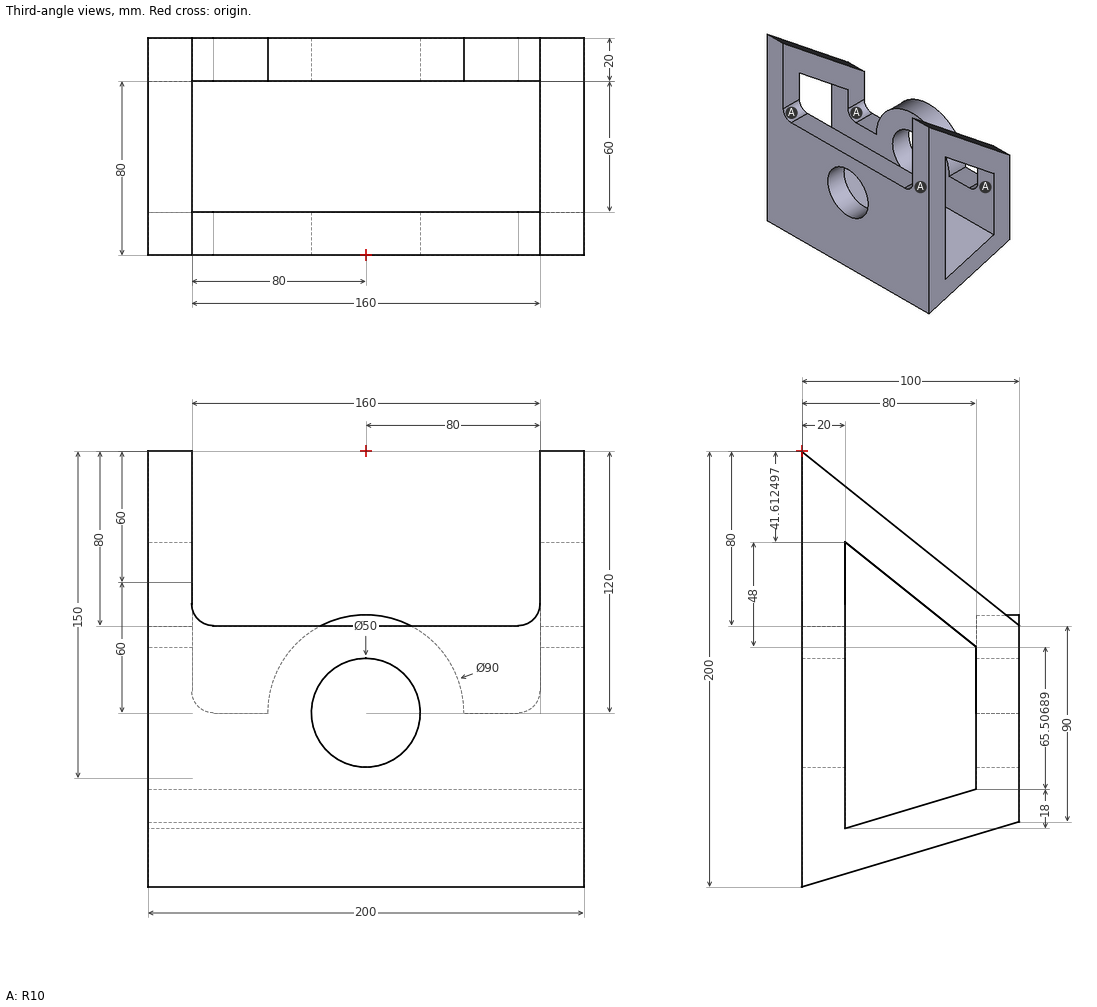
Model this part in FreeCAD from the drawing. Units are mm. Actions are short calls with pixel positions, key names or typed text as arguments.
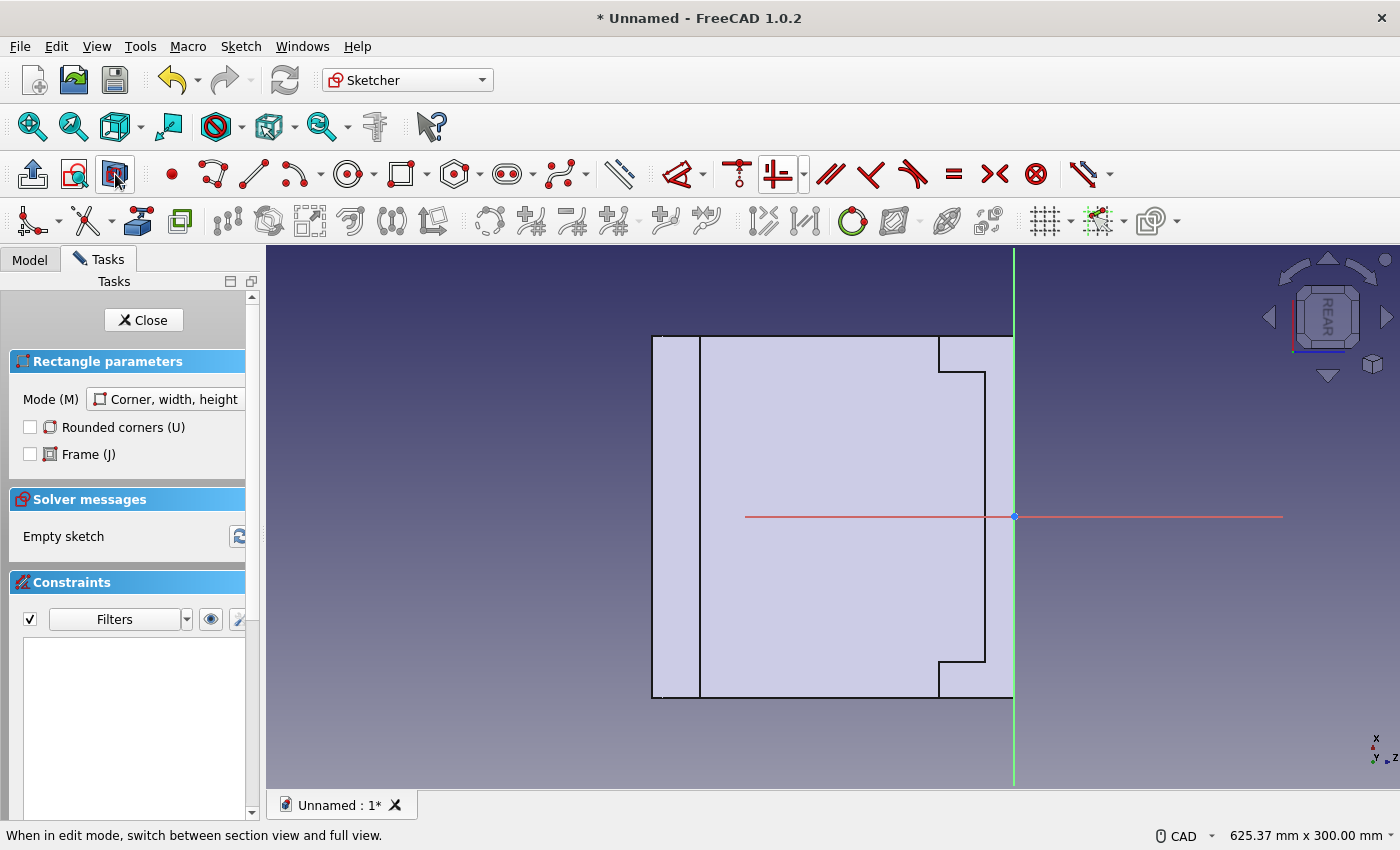
click(869, 372)
click(1014, 662)
key(Escape)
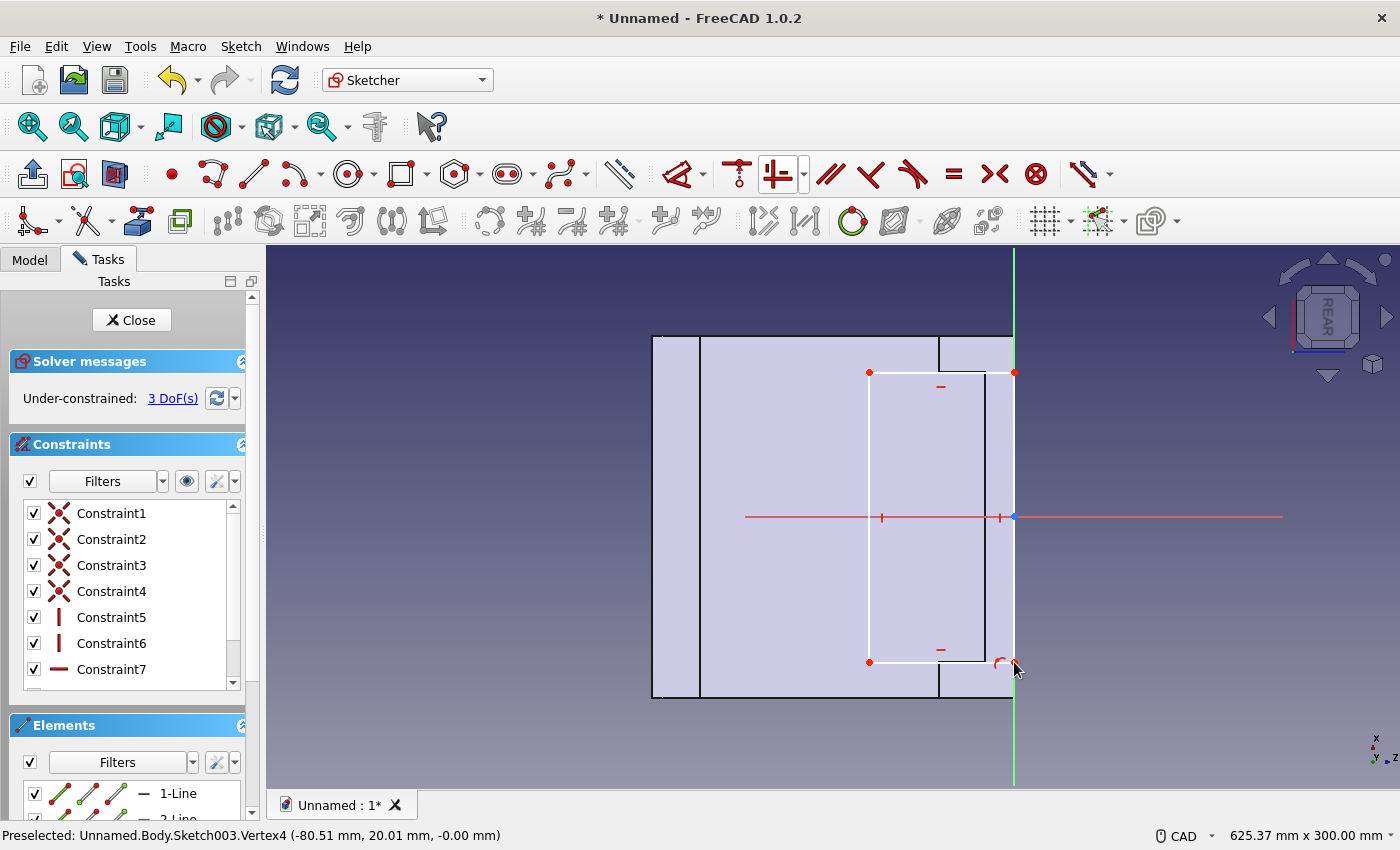
click(676, 174)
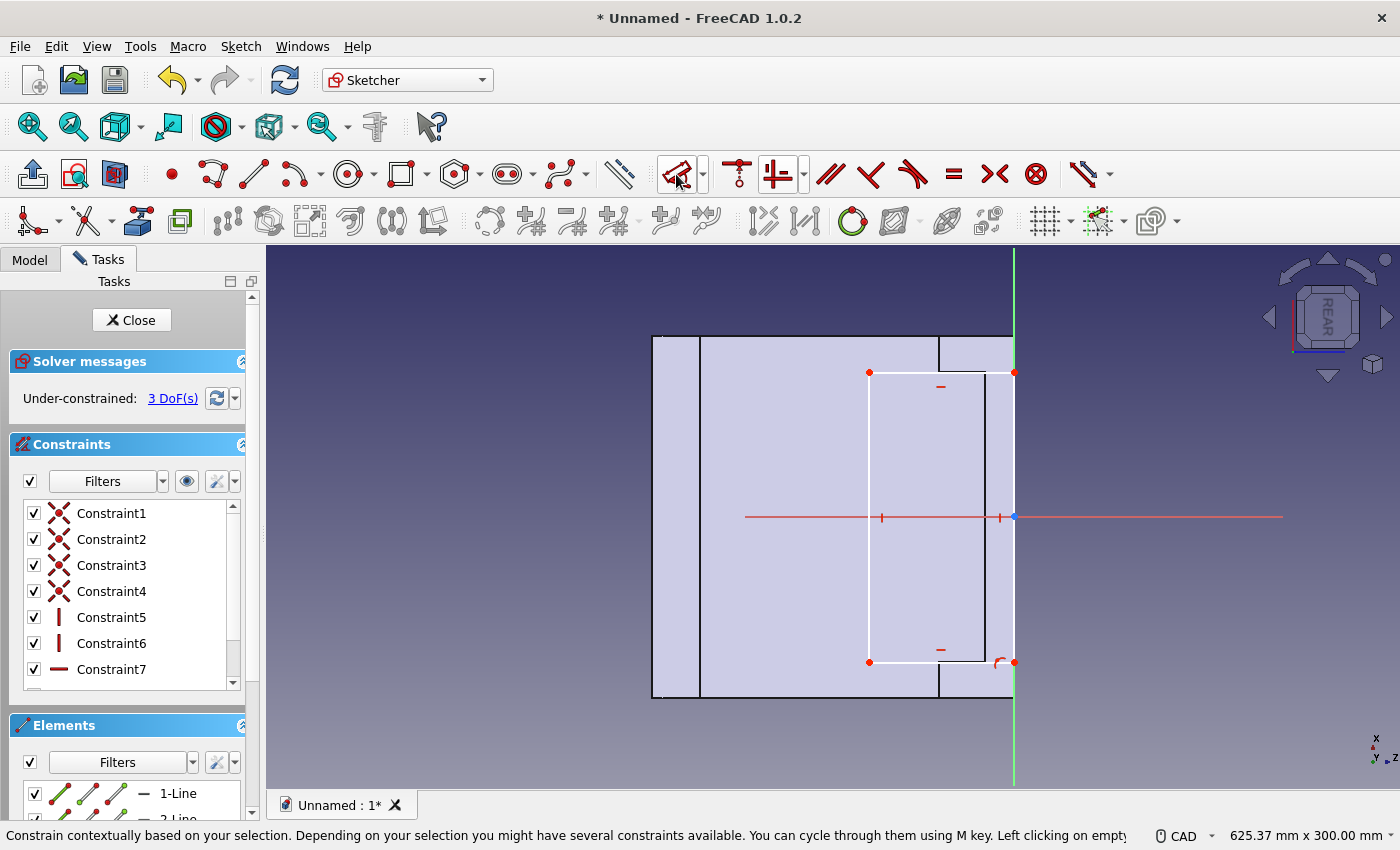
click(913, 663)
click(942, 697)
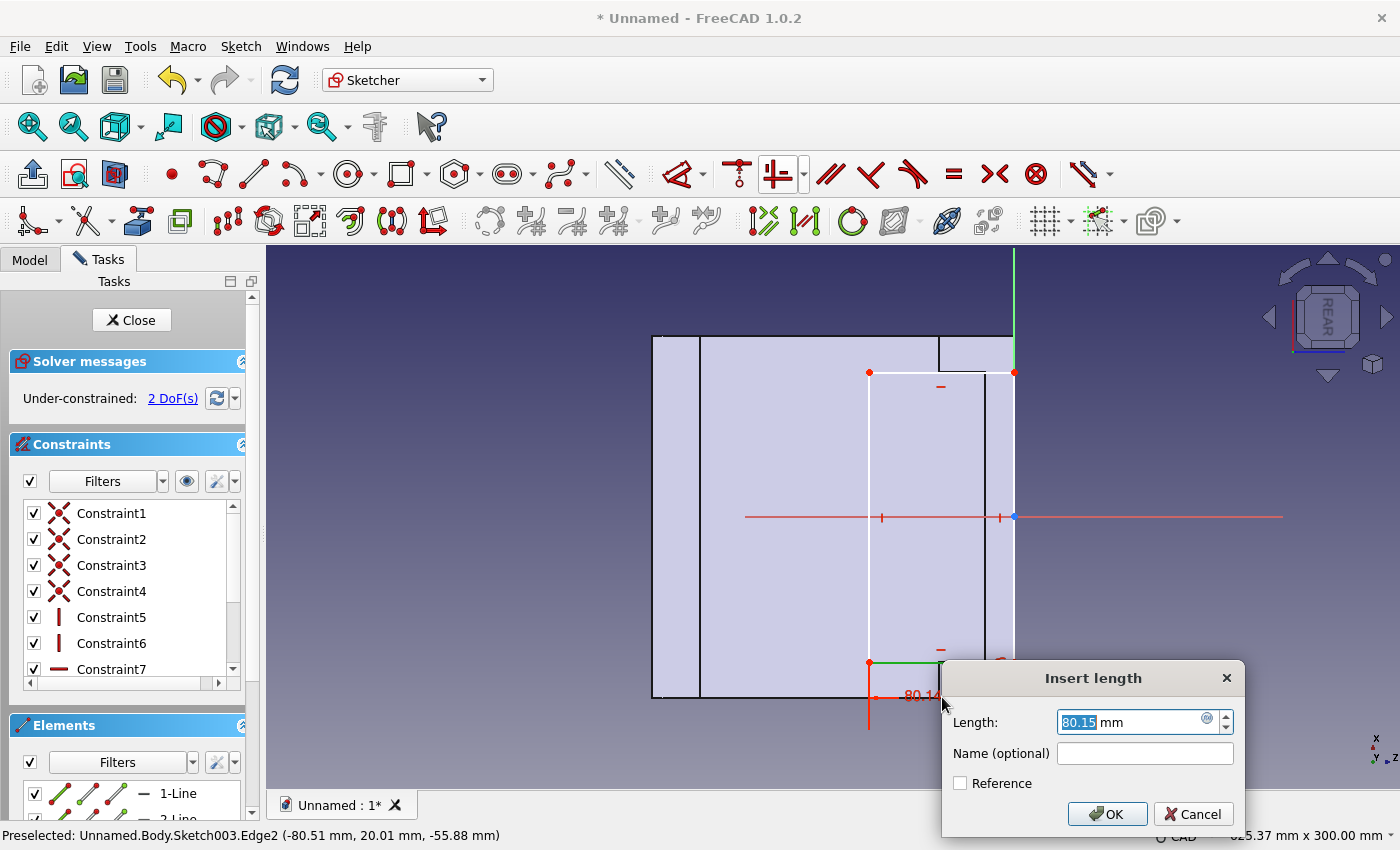
text(80)
key(Return)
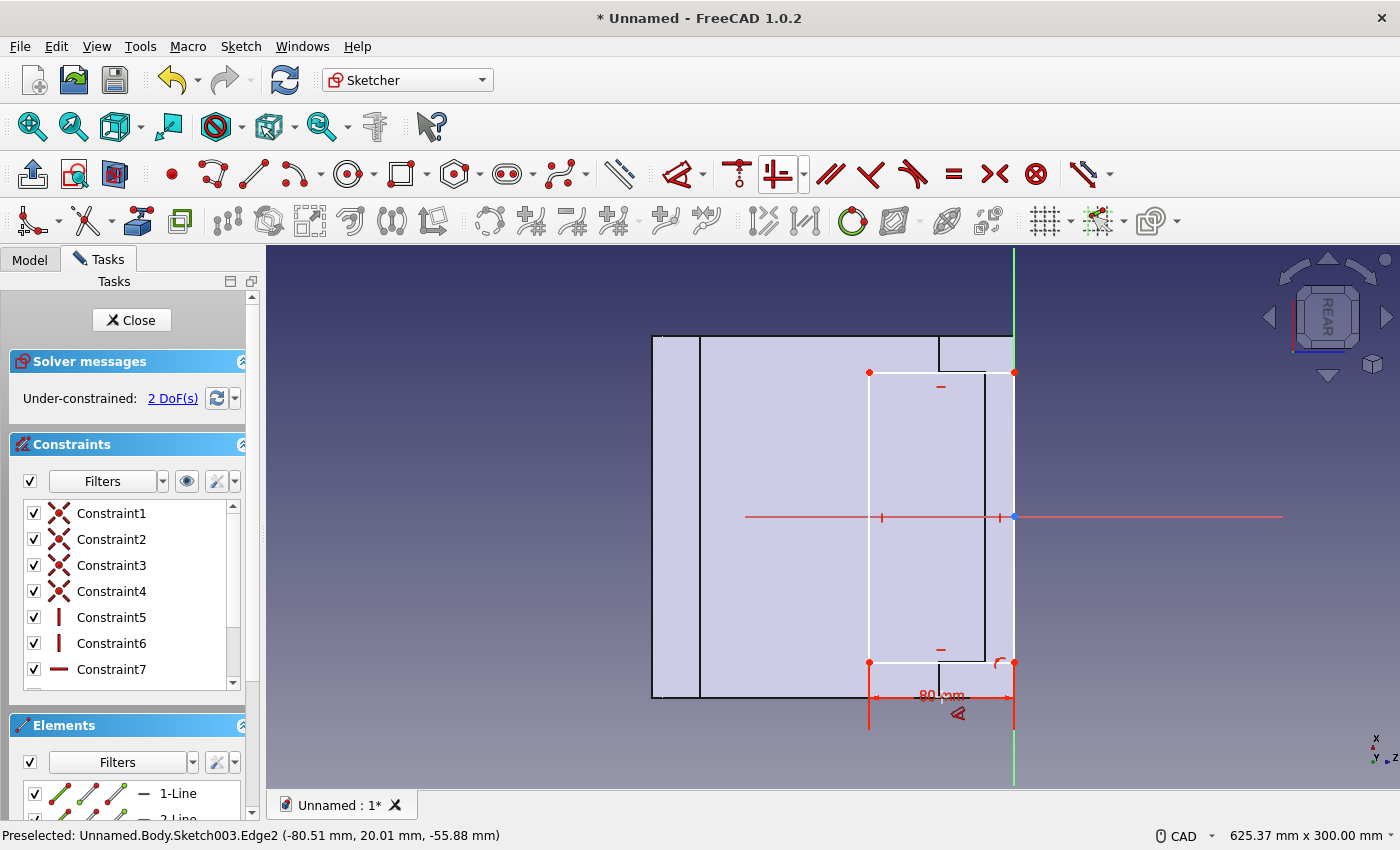
click(869, 460)
click(835, 451)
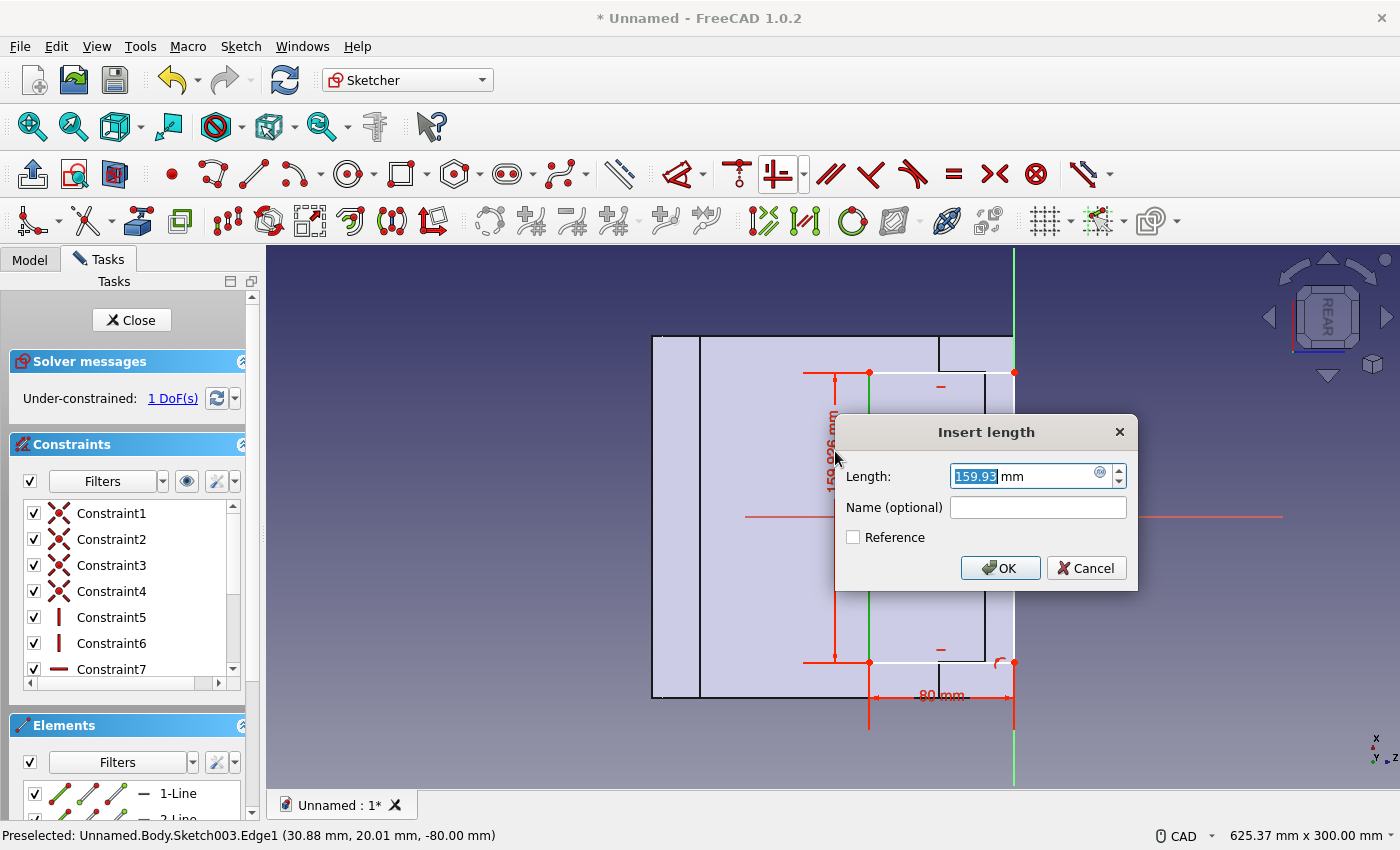
text(160)
key(Return)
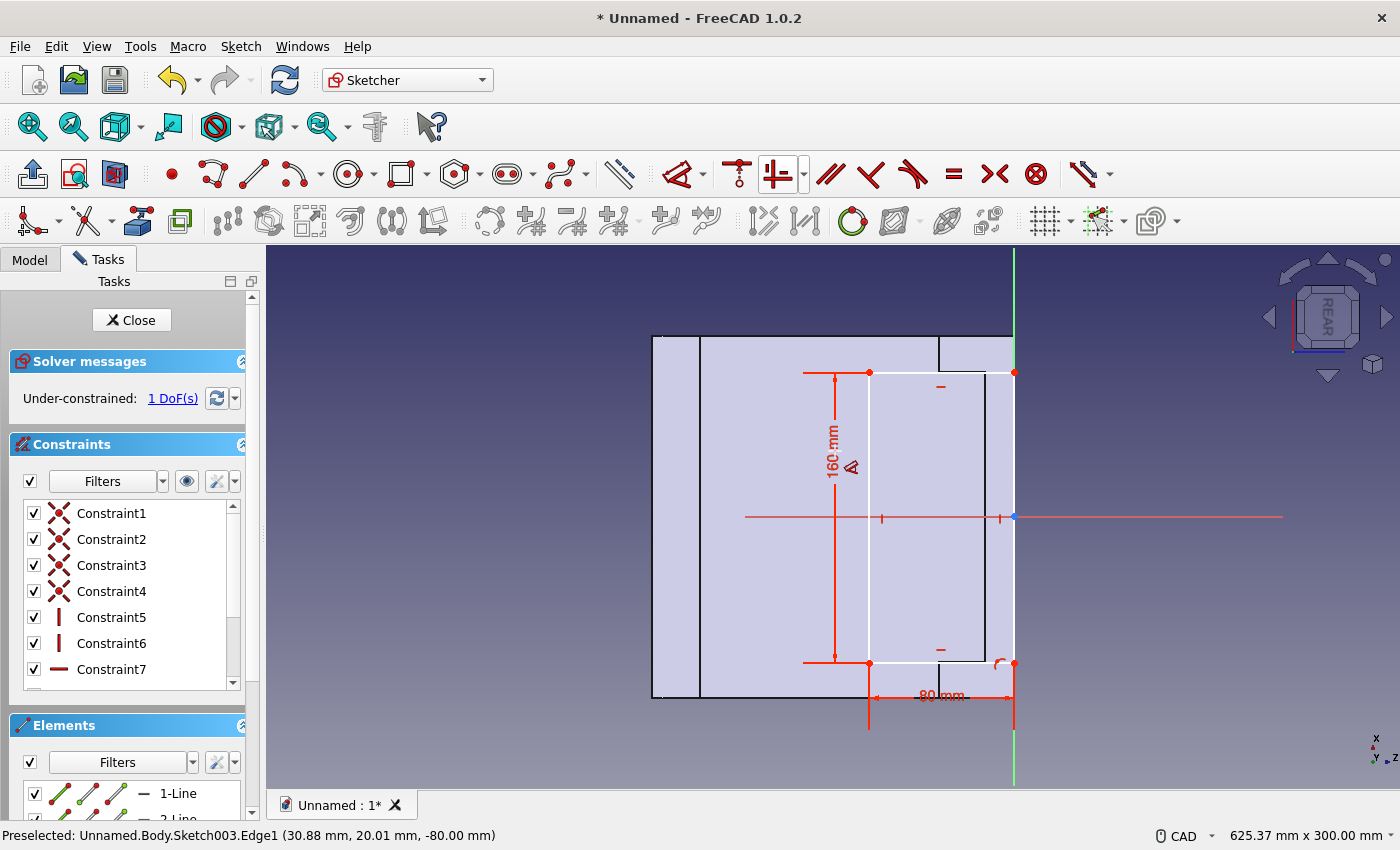
click(869, 373)
click(1048, 445)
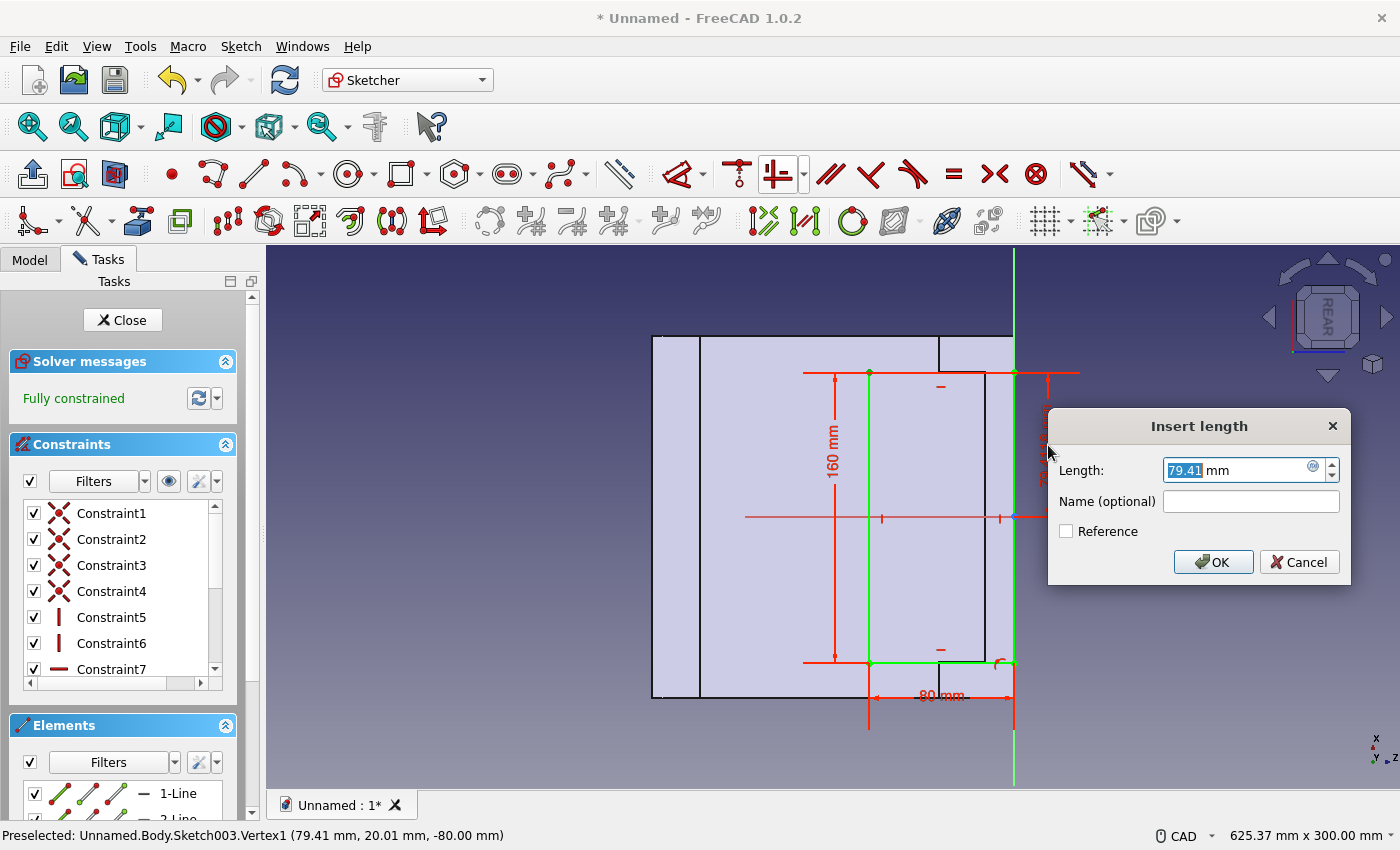
text(80)
key(Return)
key(Escape)